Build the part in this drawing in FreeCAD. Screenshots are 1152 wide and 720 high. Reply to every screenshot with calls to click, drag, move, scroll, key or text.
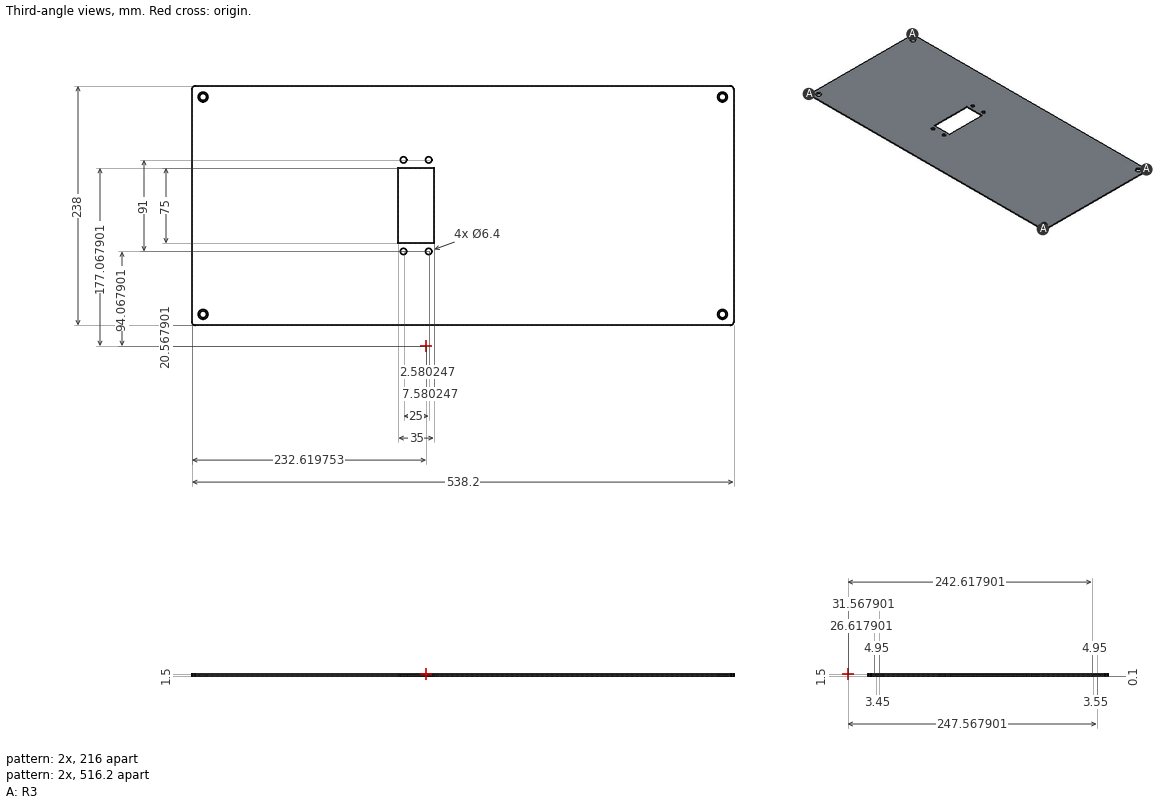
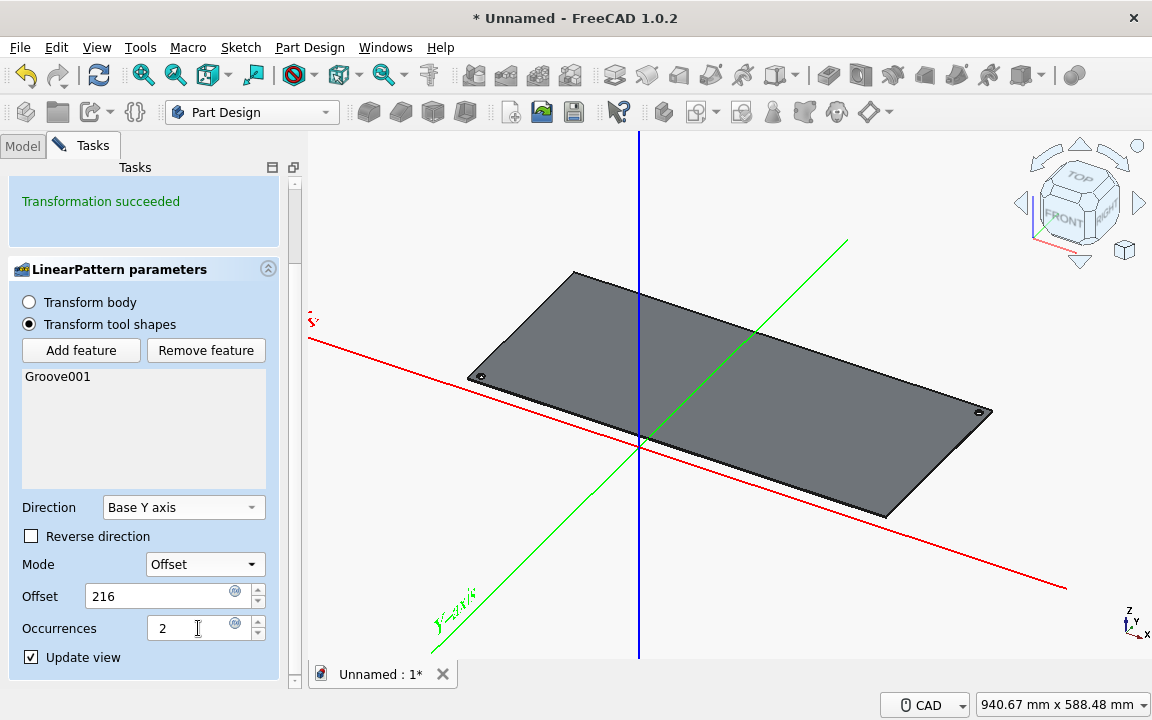
click(30, 536)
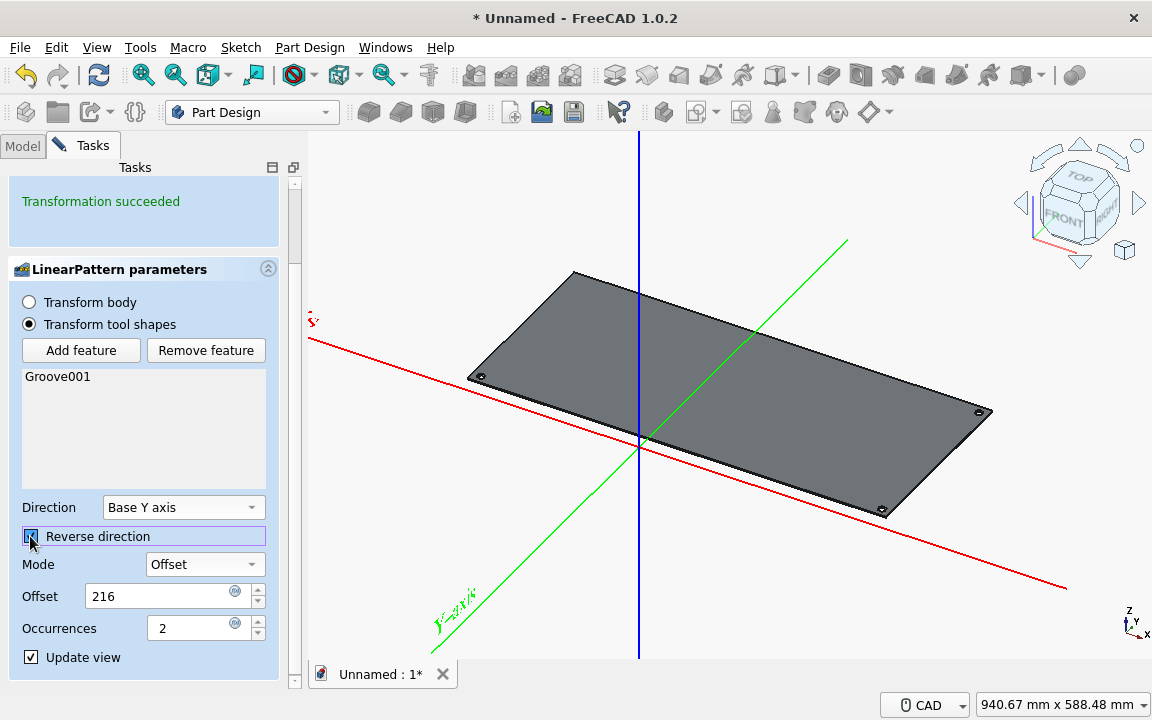
scroll(295, 432, up, 3)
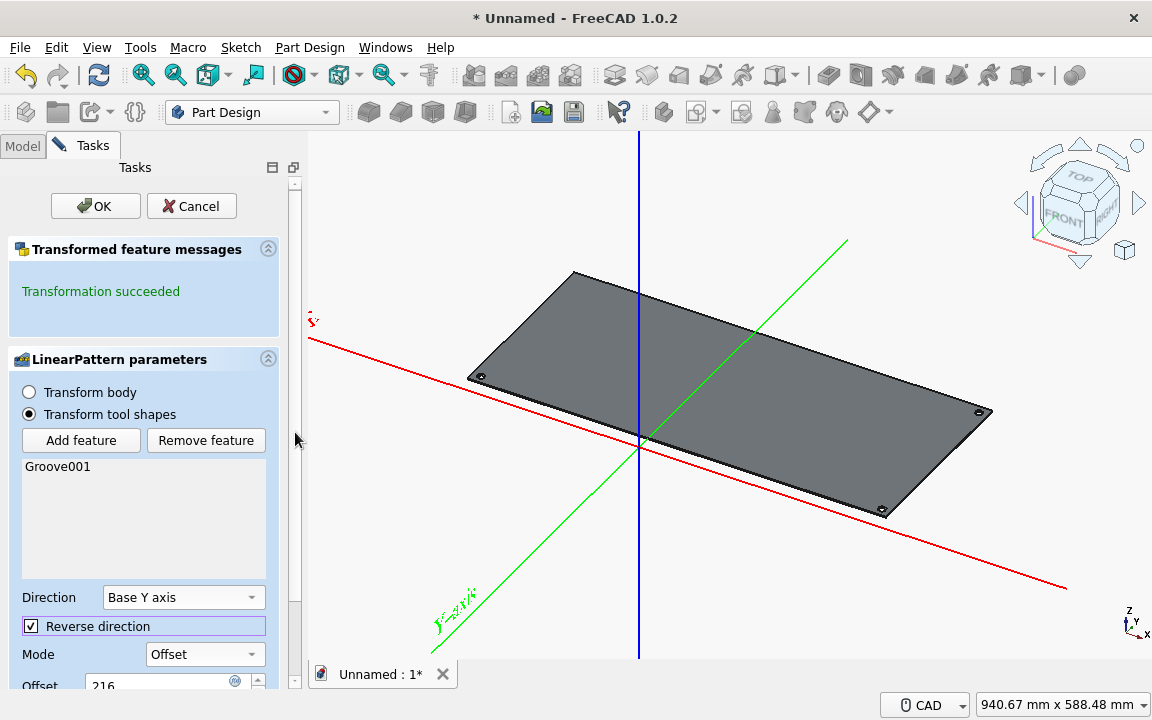
click(96, 206)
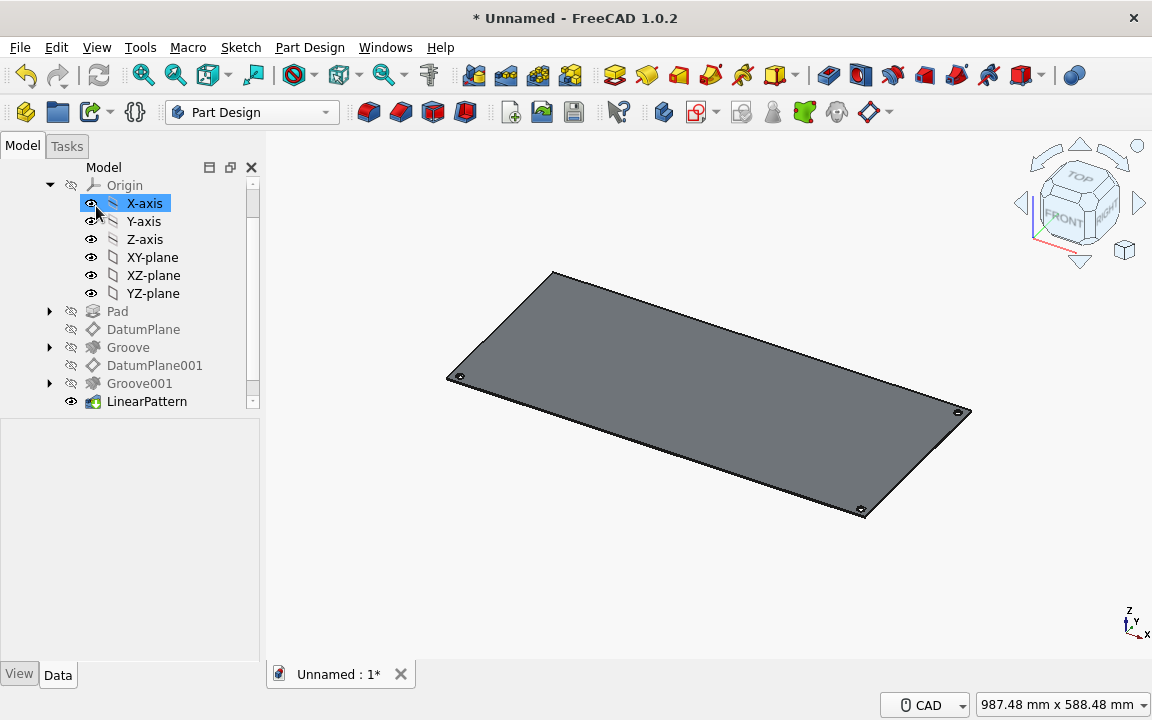
click(116, 383)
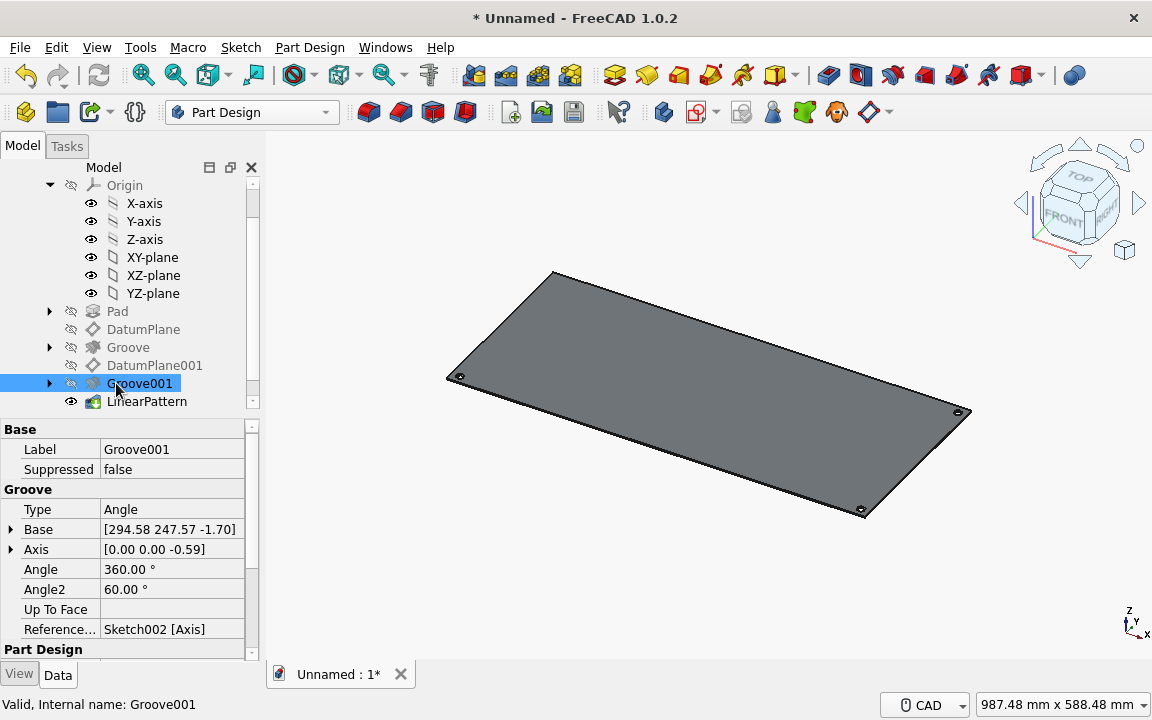
click(506, 76)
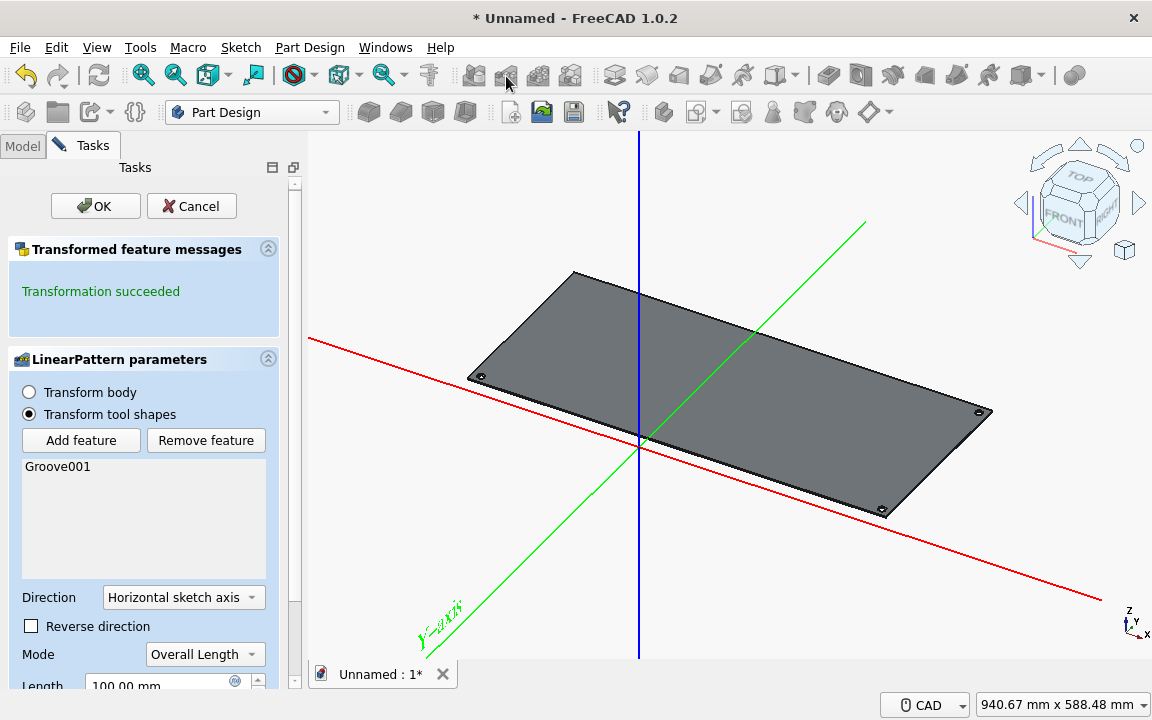
click(184, 598)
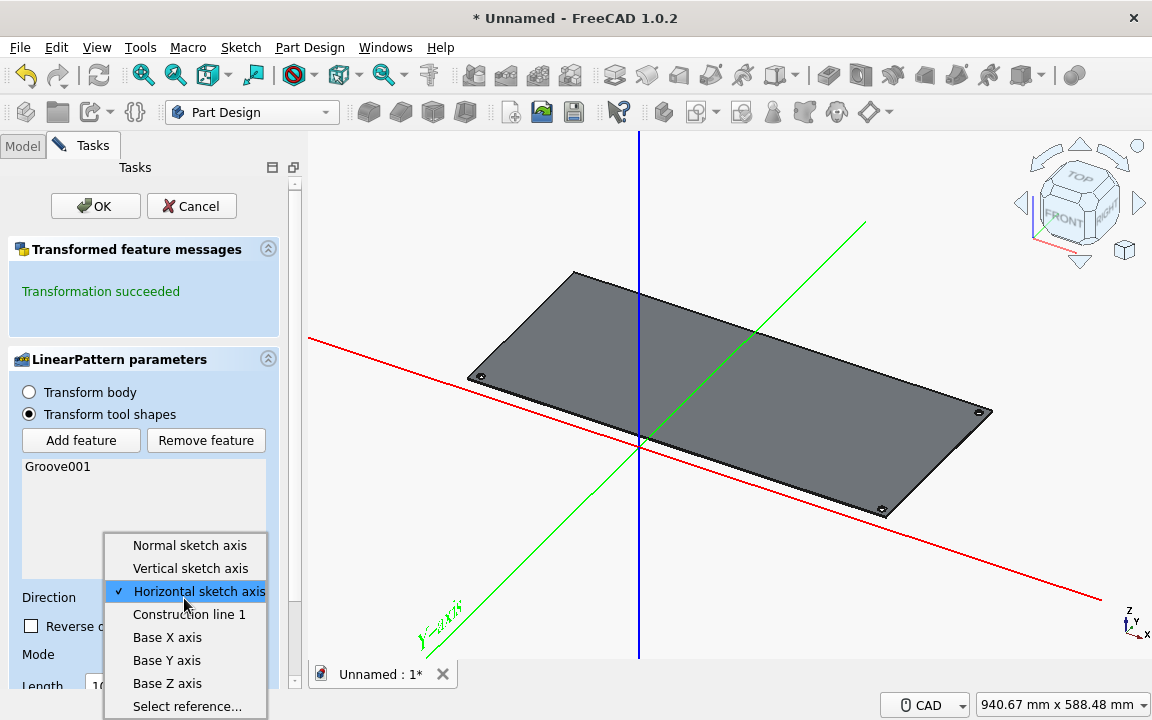
click(184, 638)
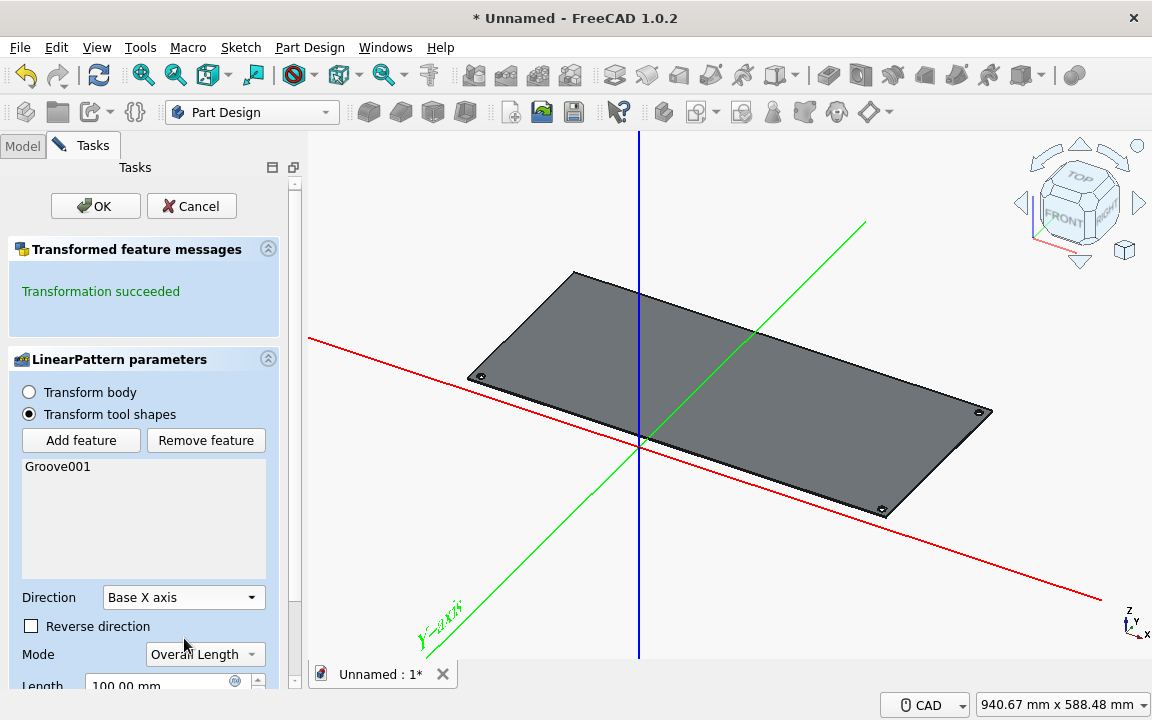
click(206, 654)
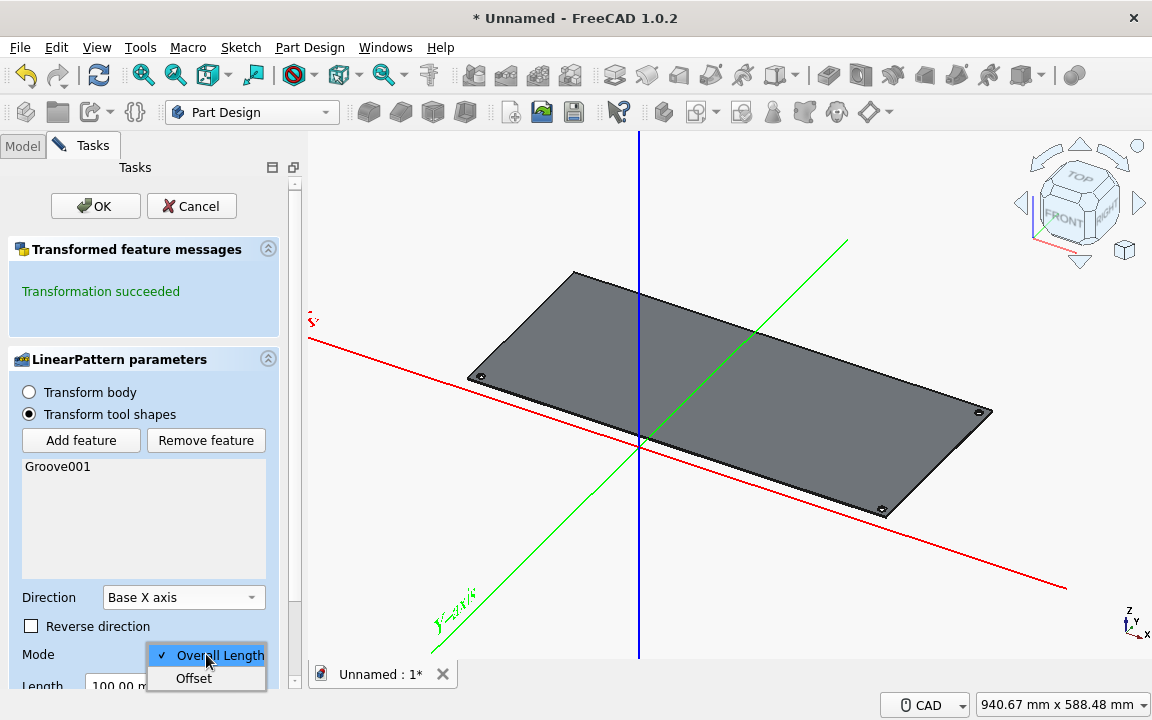
click(206, 678)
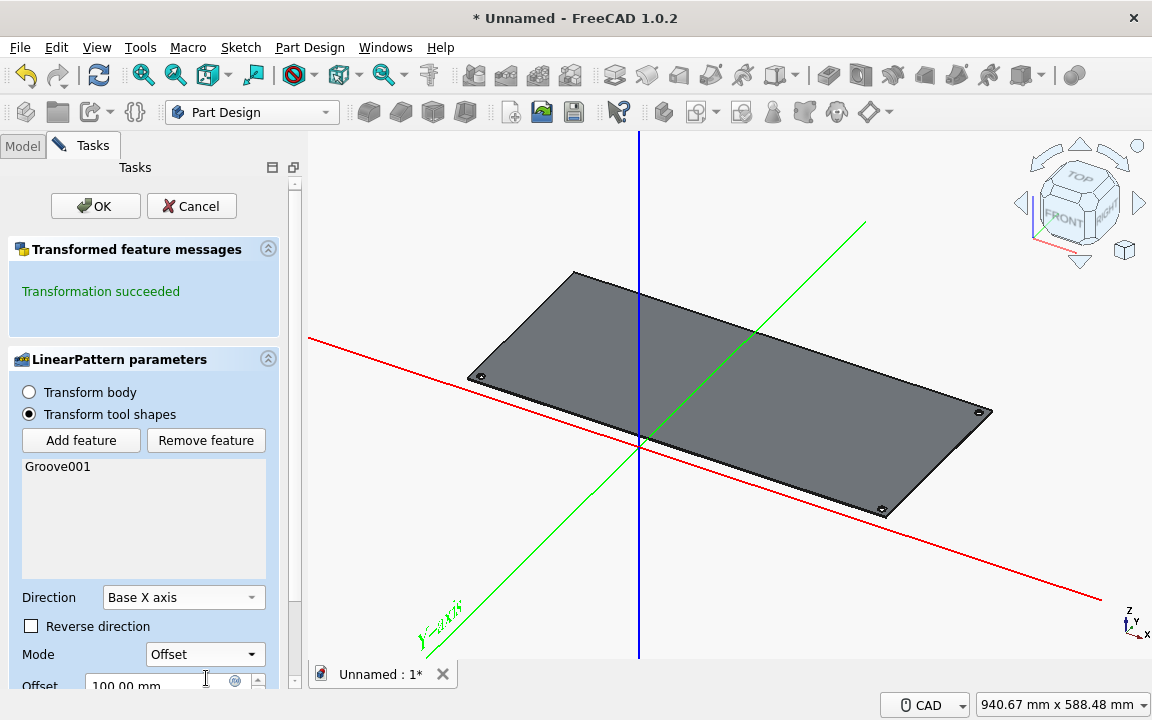
scroll(295, 432, down, 2)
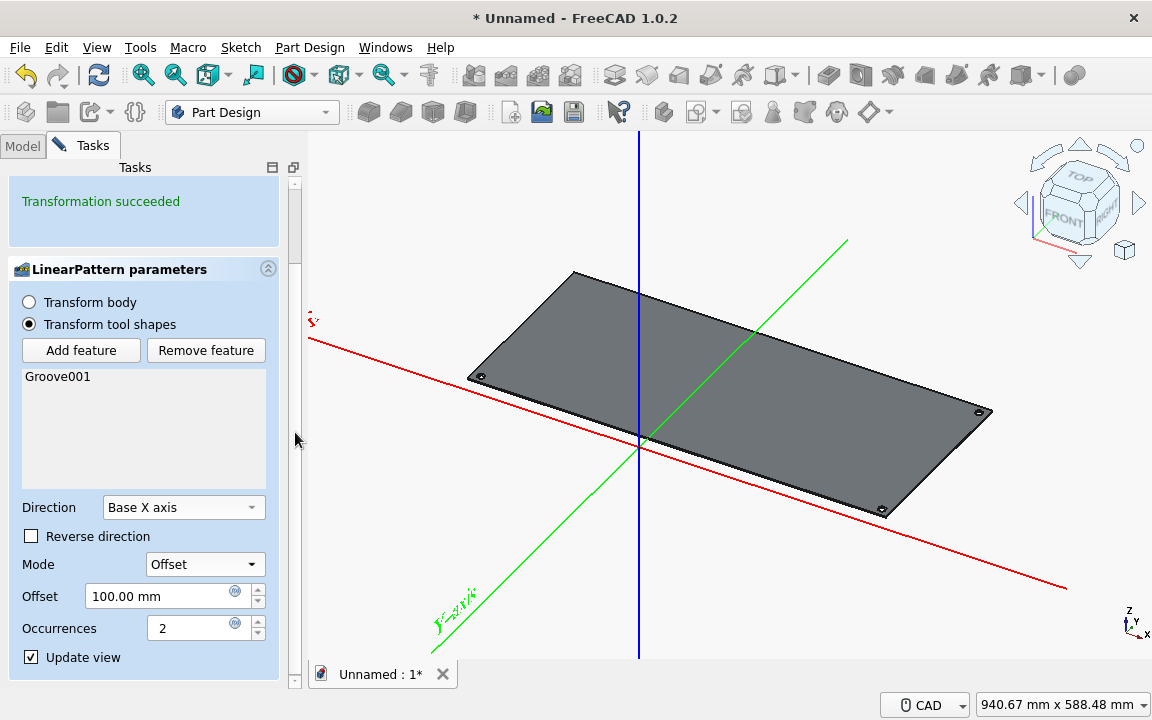
triple_click(168, 596)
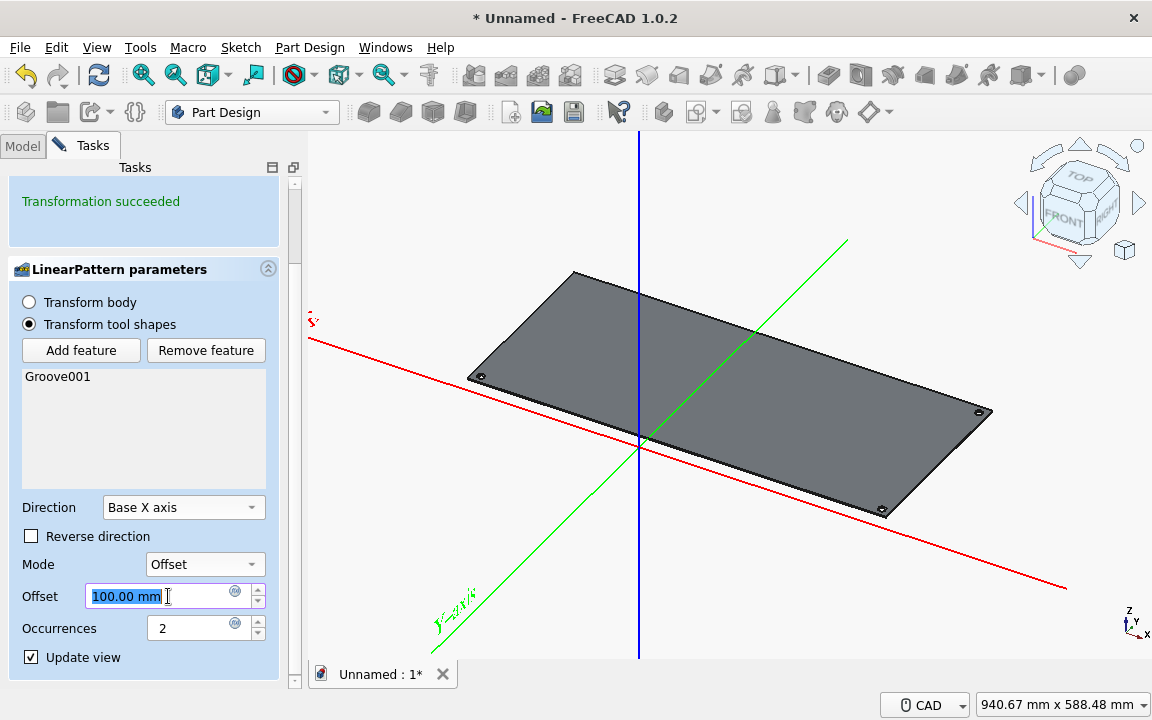
text(516.2)
key(Tab)